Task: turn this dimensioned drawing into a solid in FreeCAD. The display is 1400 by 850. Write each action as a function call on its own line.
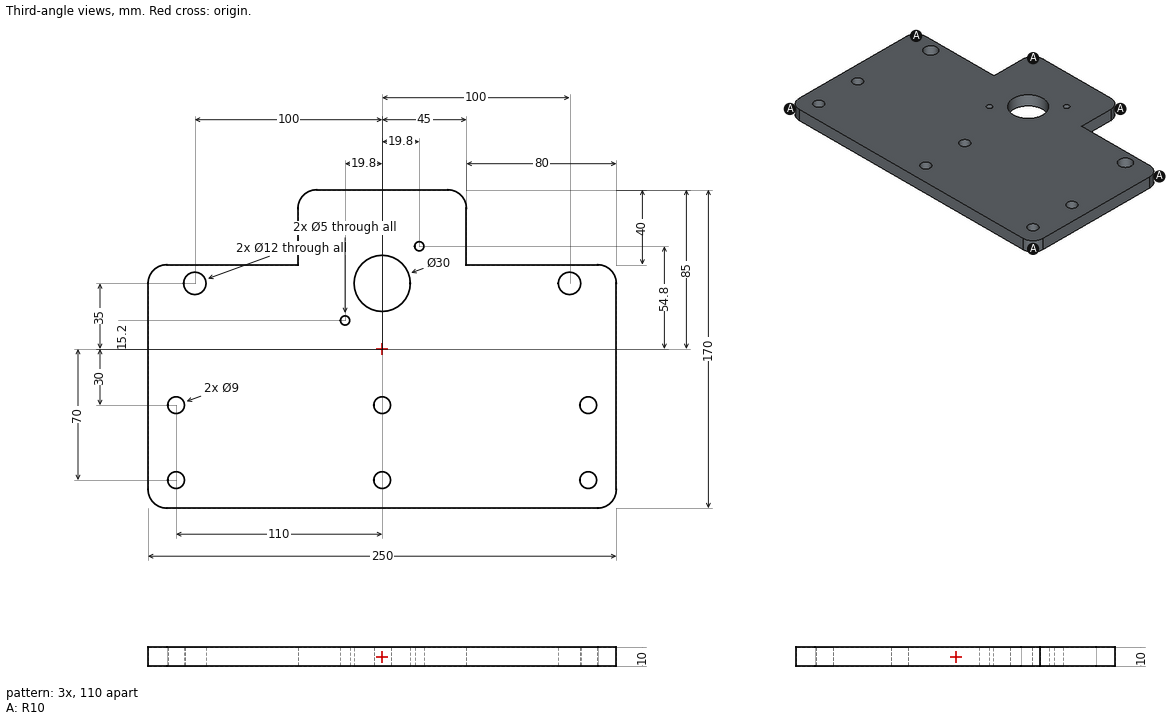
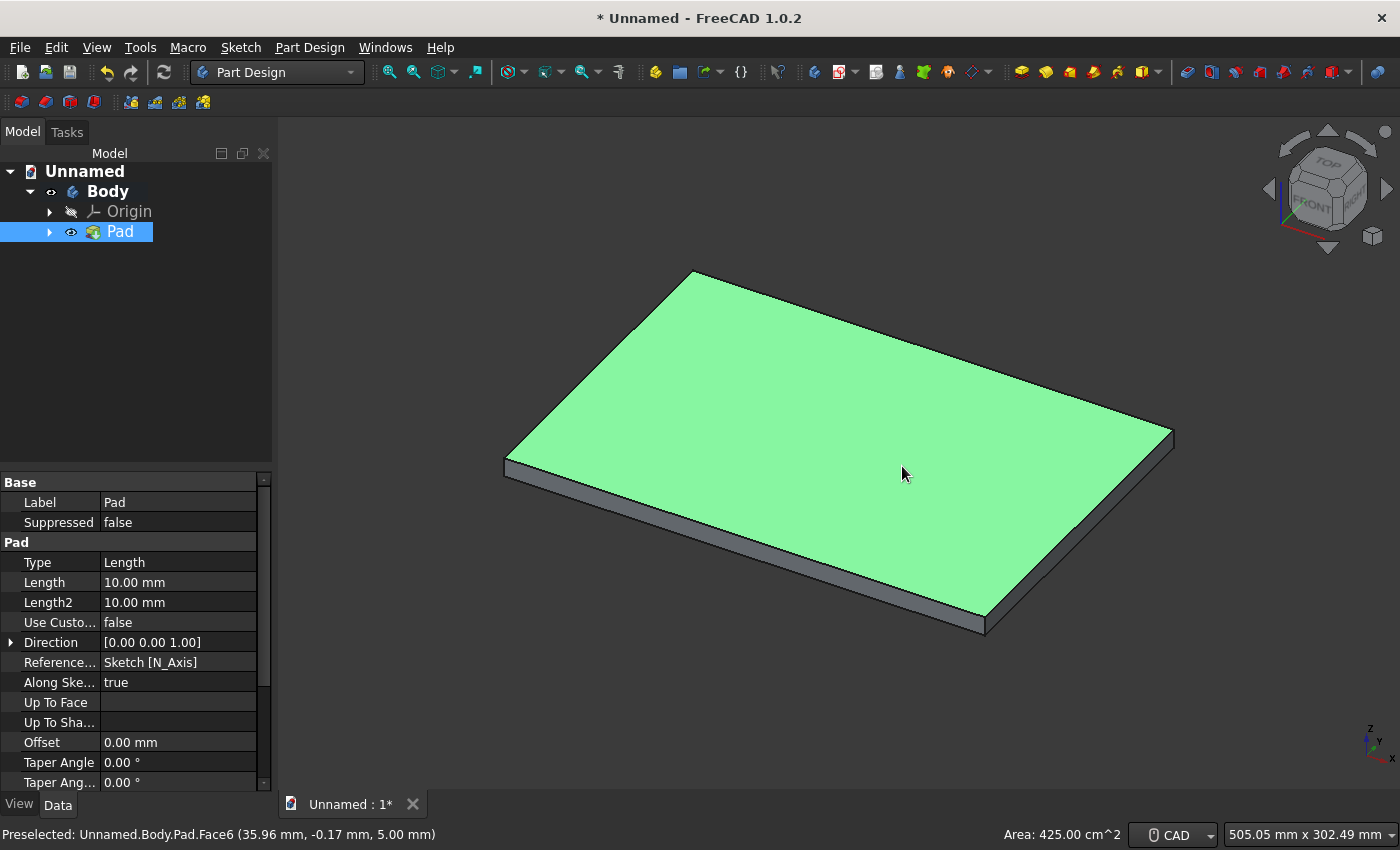
click(840, 72)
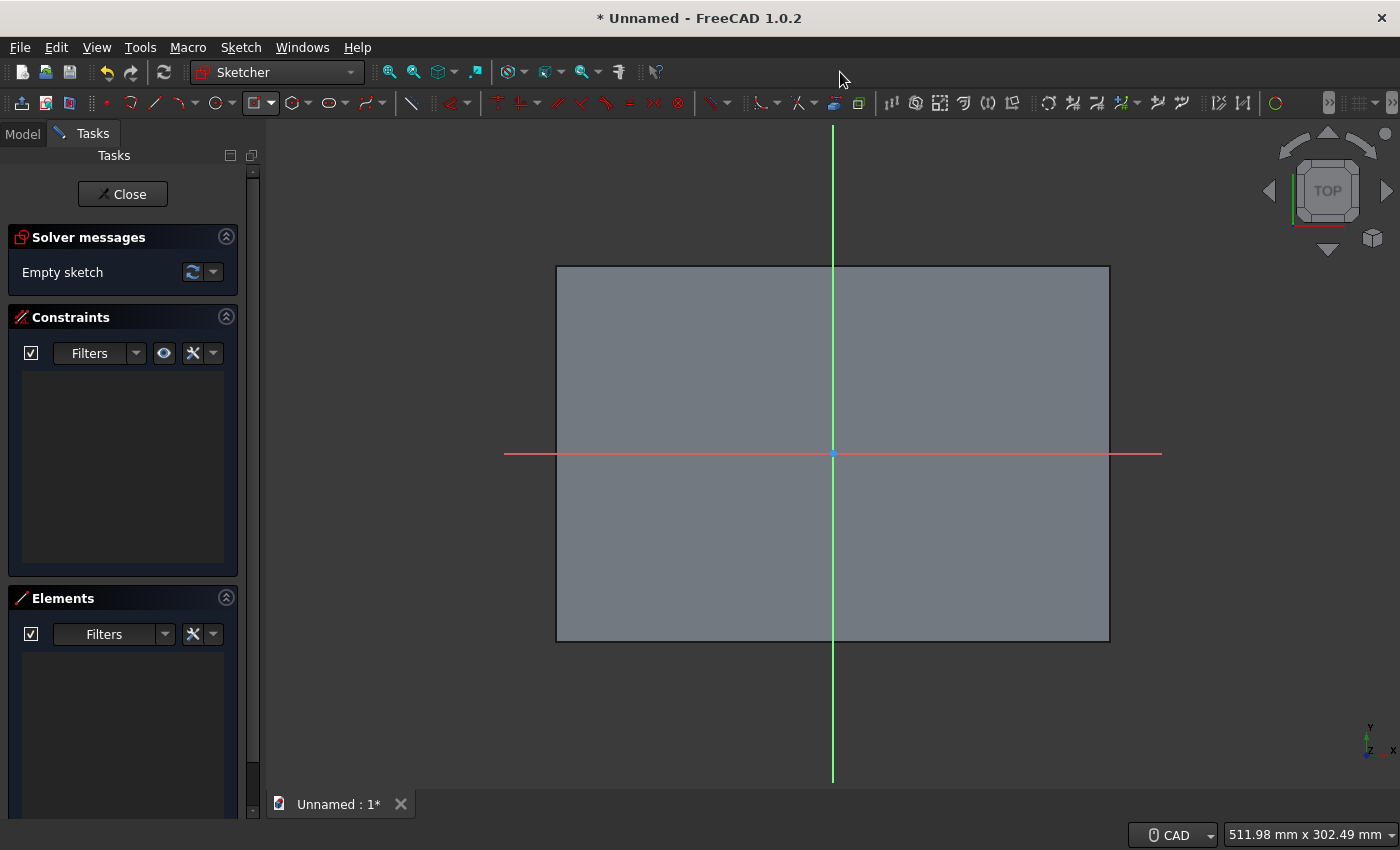
scroll(1140, 283, up, 4)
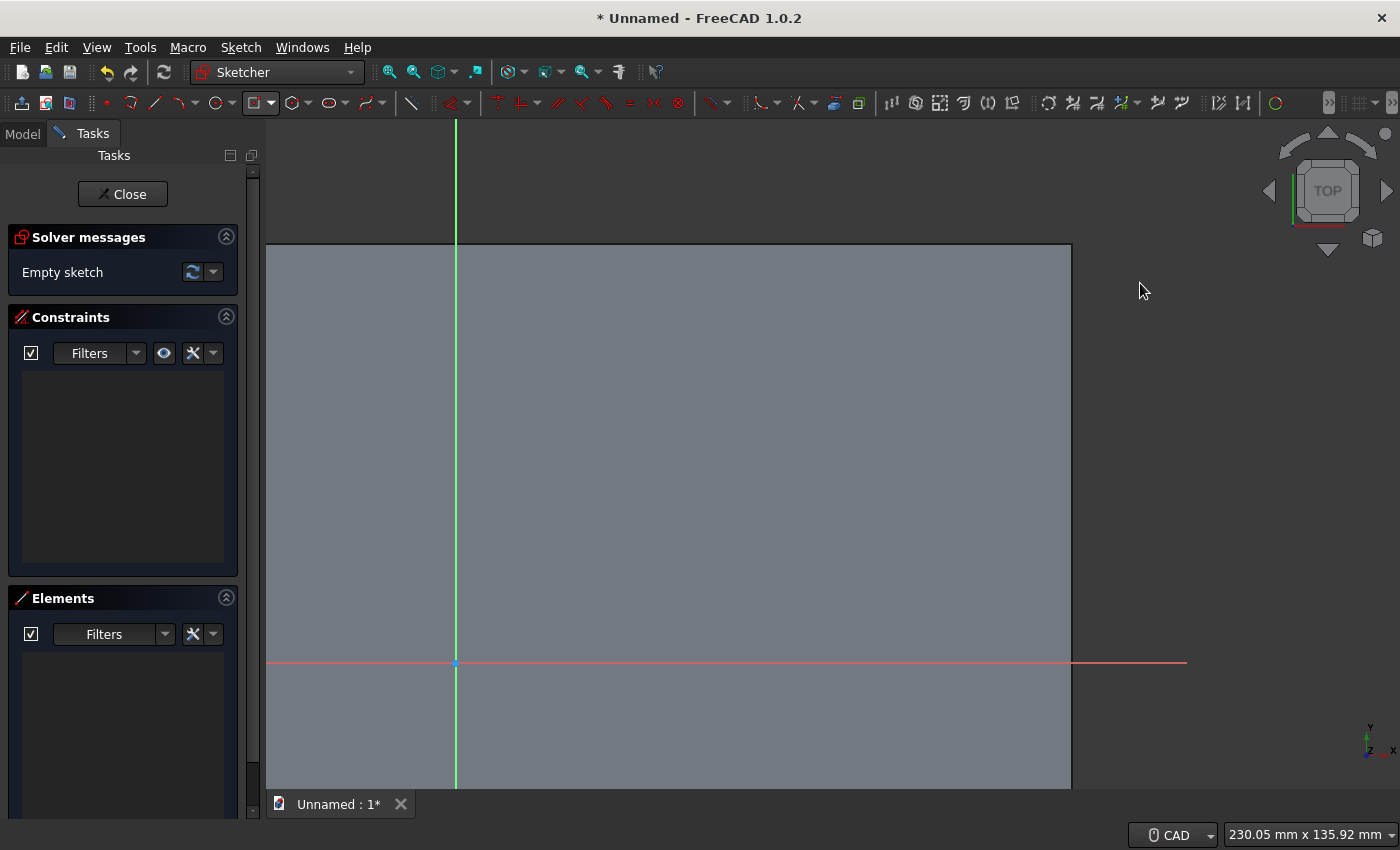
key(g)
key(r)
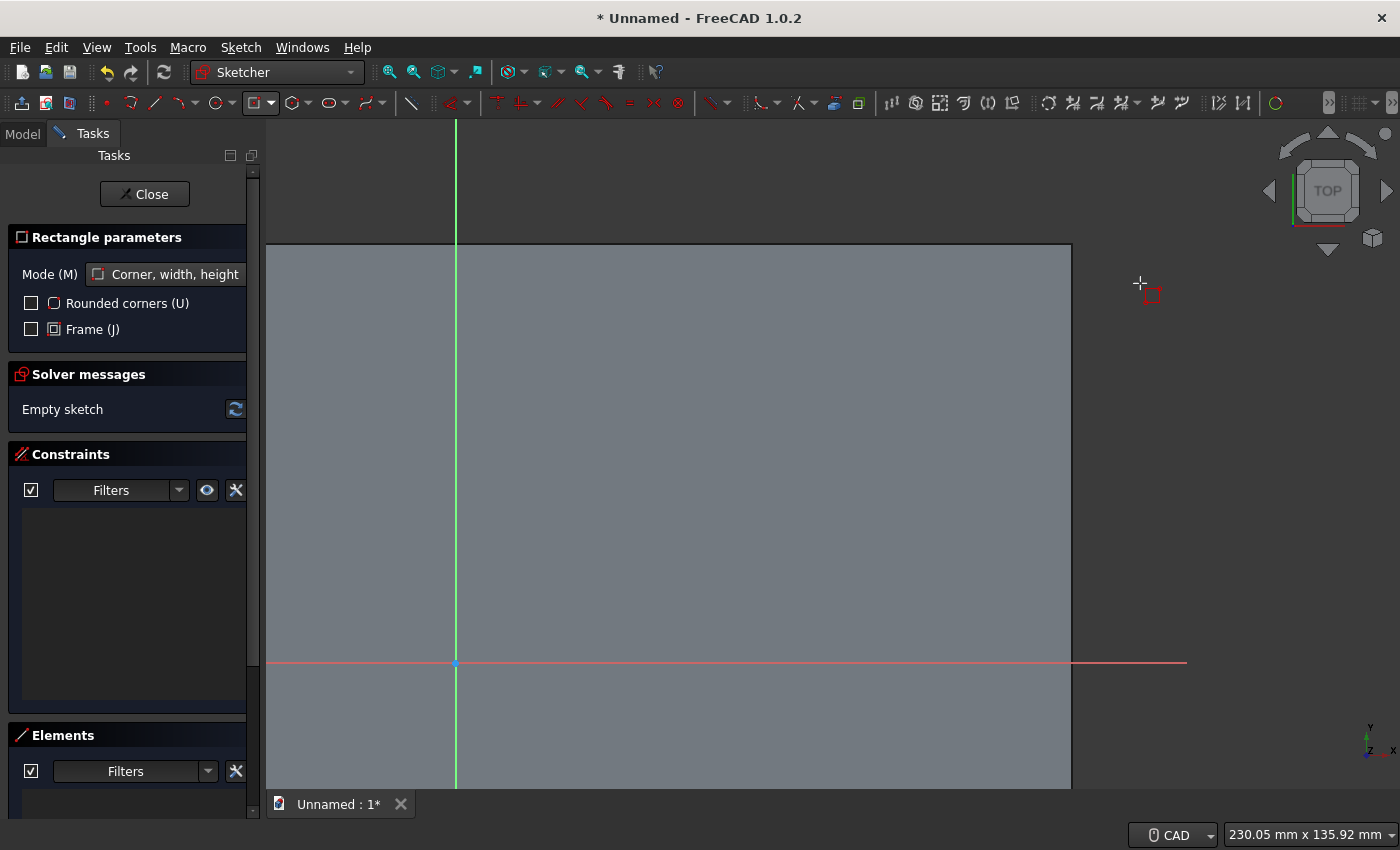
click(678, 244)
move(1072, 441)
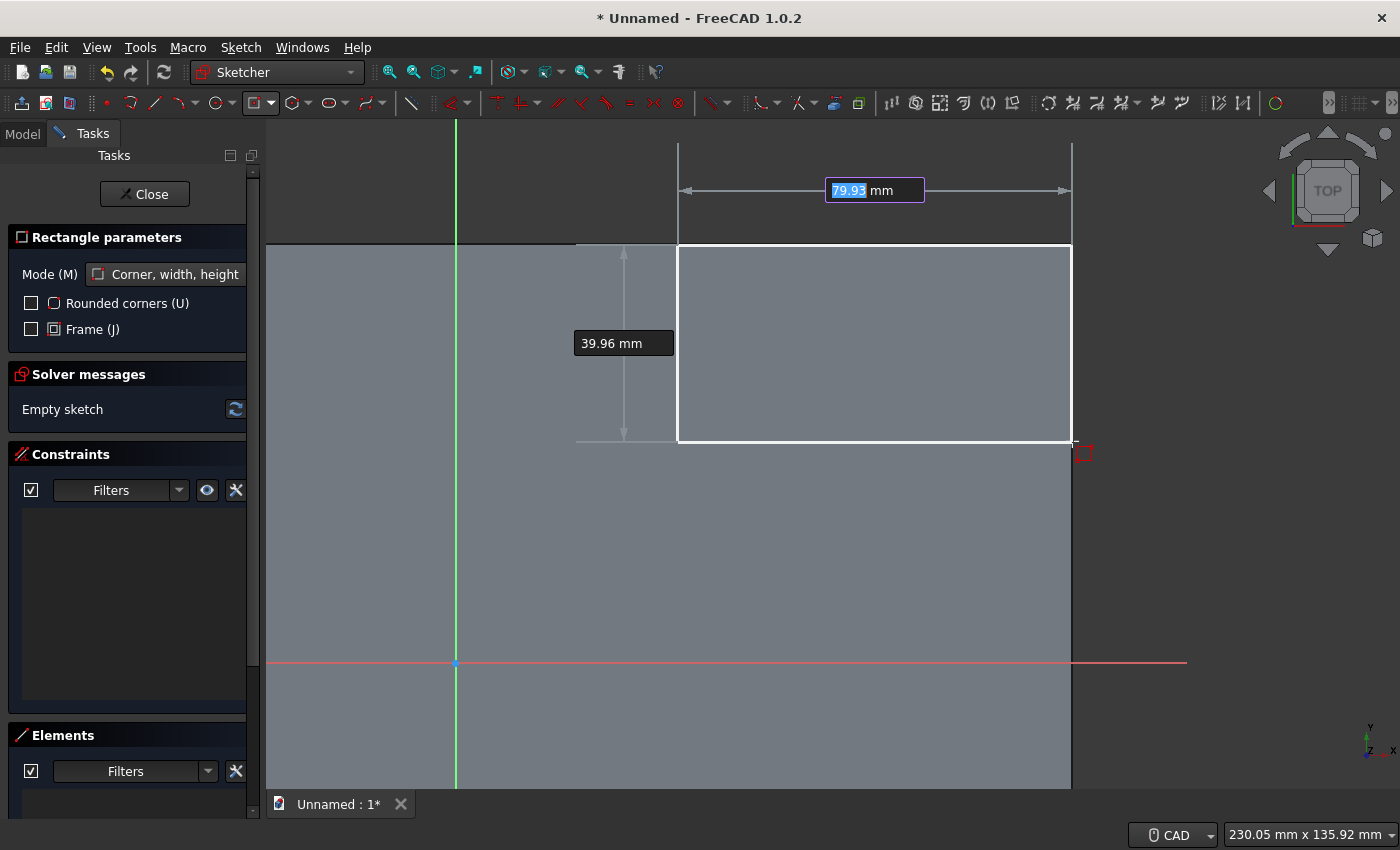
text(80)
key(Tab)
text(40)
key(Return)
key(Escape)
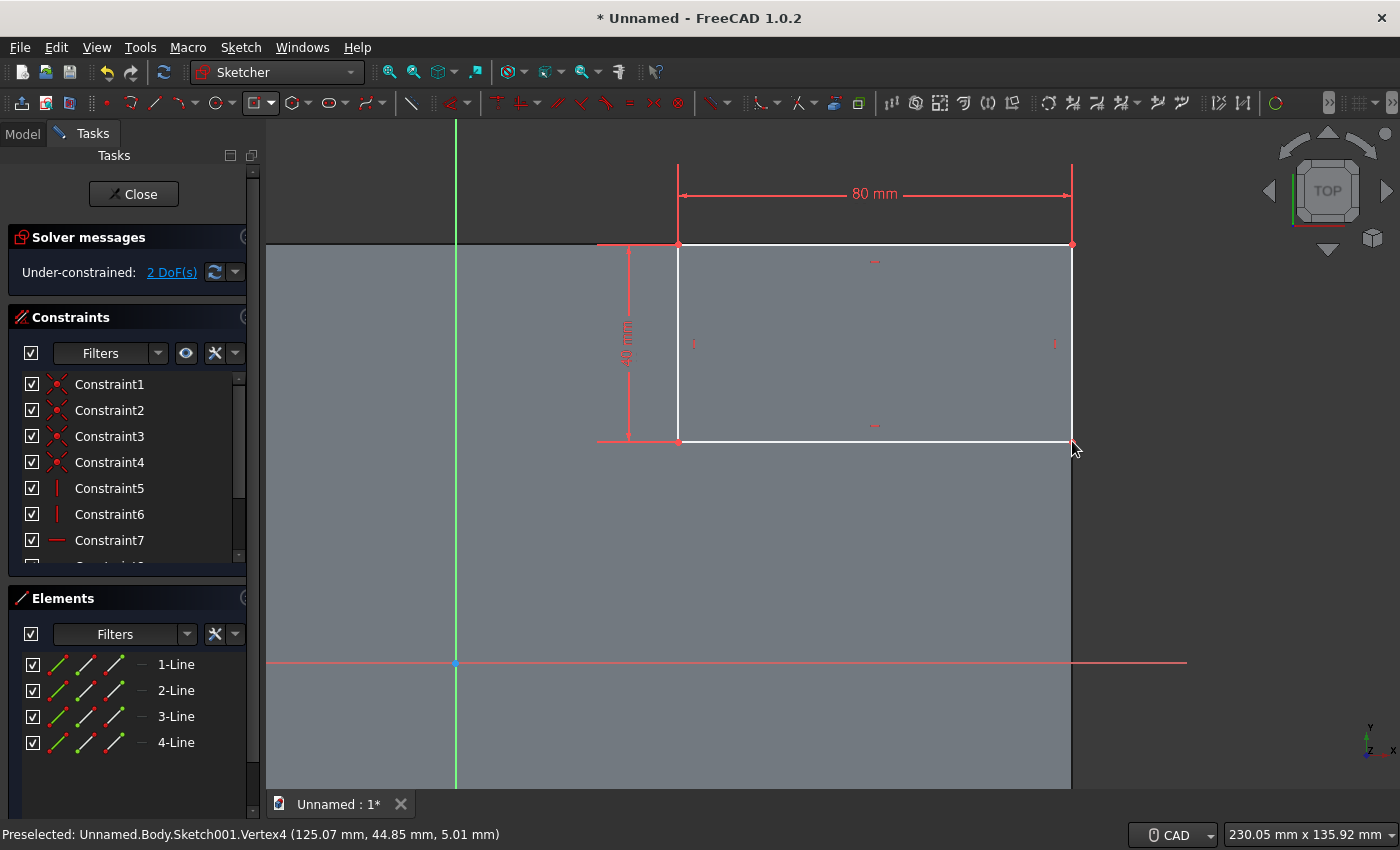
click(450, 104)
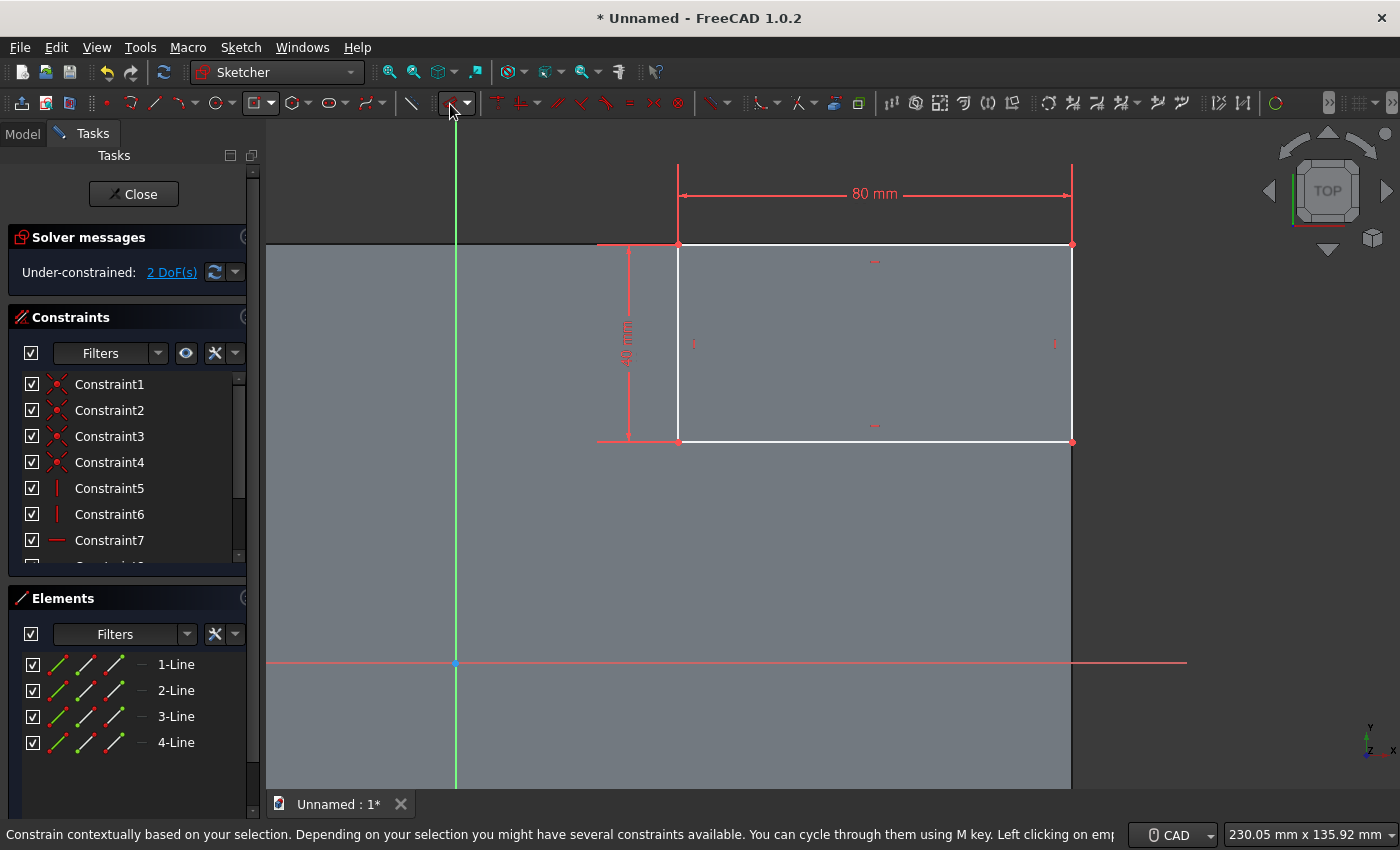
click(678, 245)
click(567, 697)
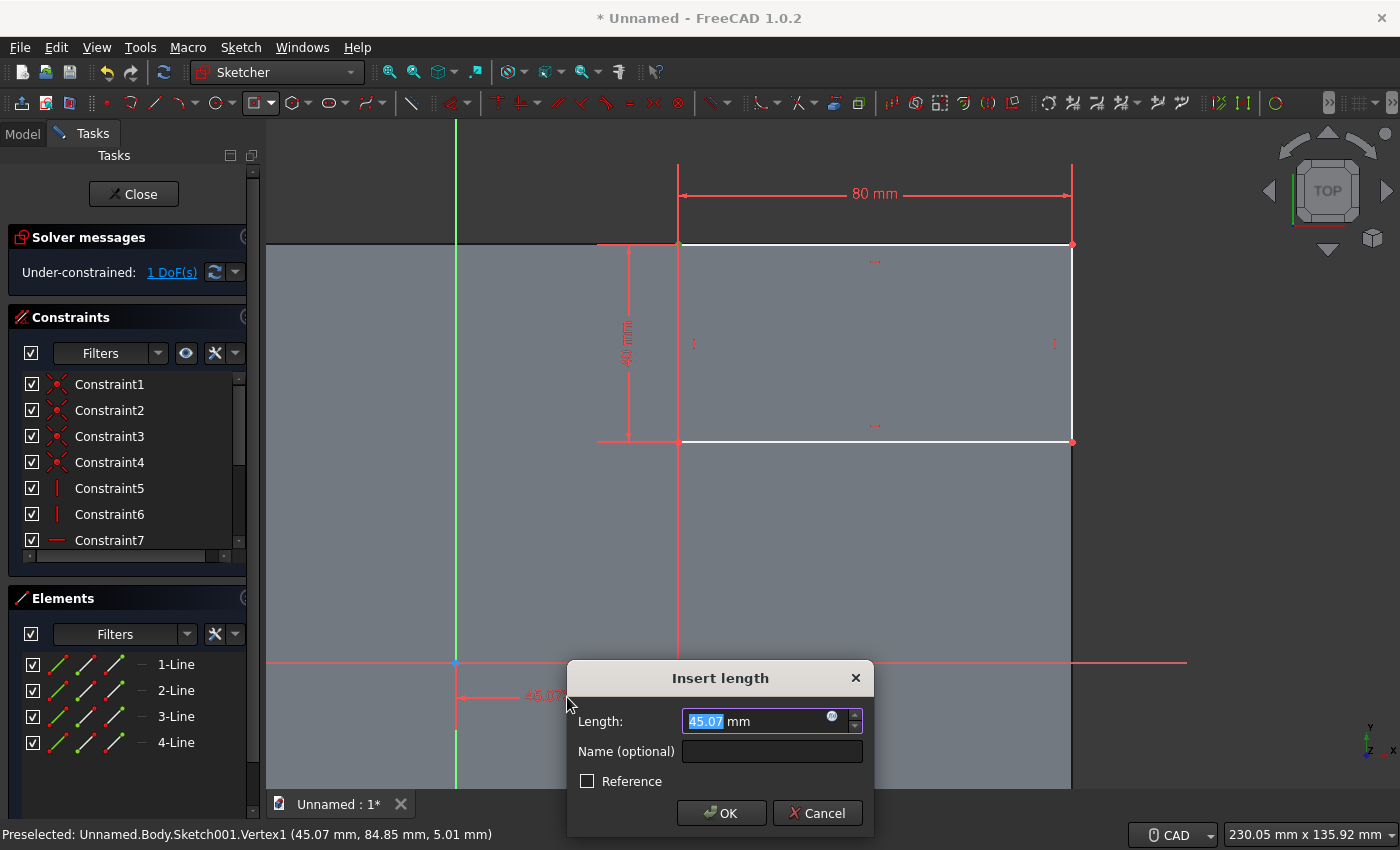
text(45)
key(Return)